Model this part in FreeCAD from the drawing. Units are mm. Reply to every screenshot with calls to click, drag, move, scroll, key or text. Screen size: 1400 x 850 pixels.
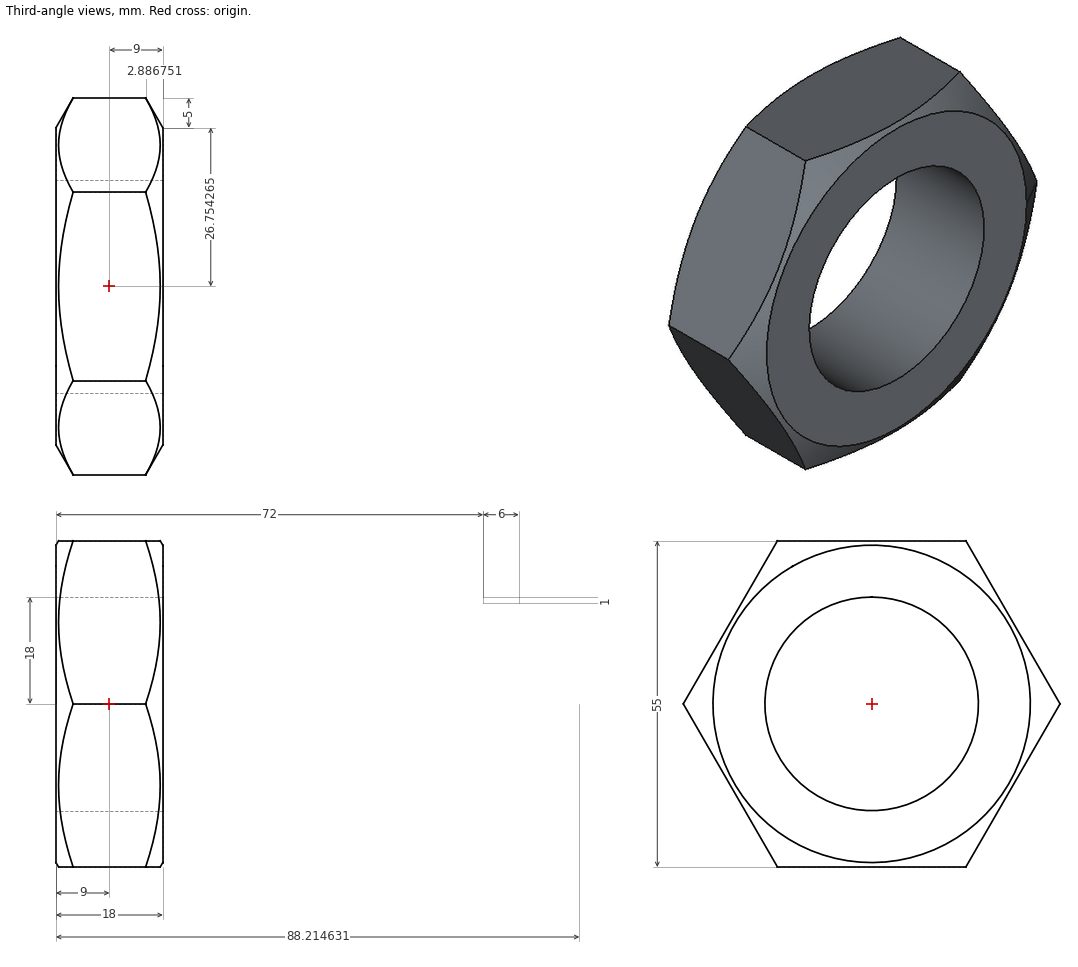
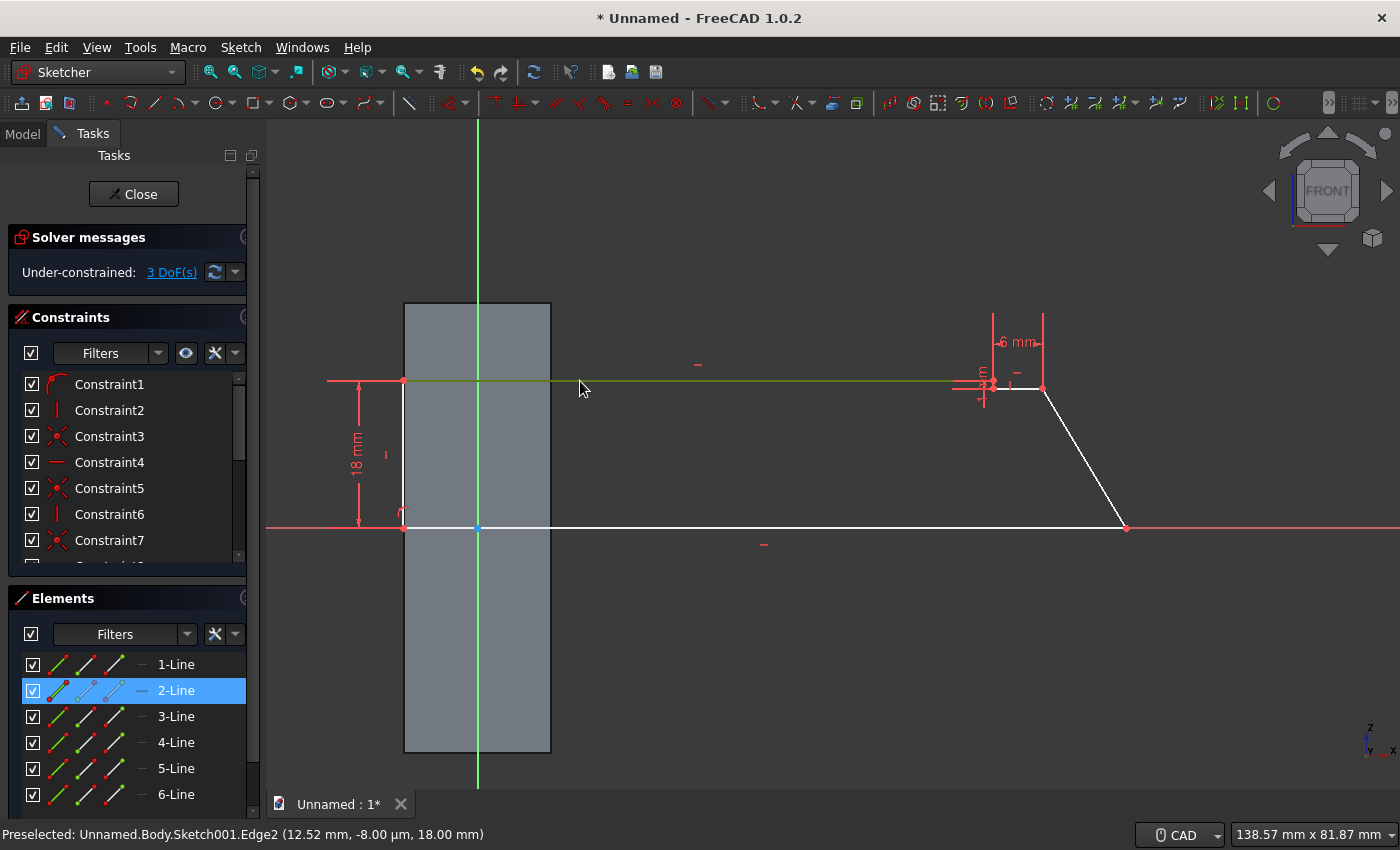
key(l)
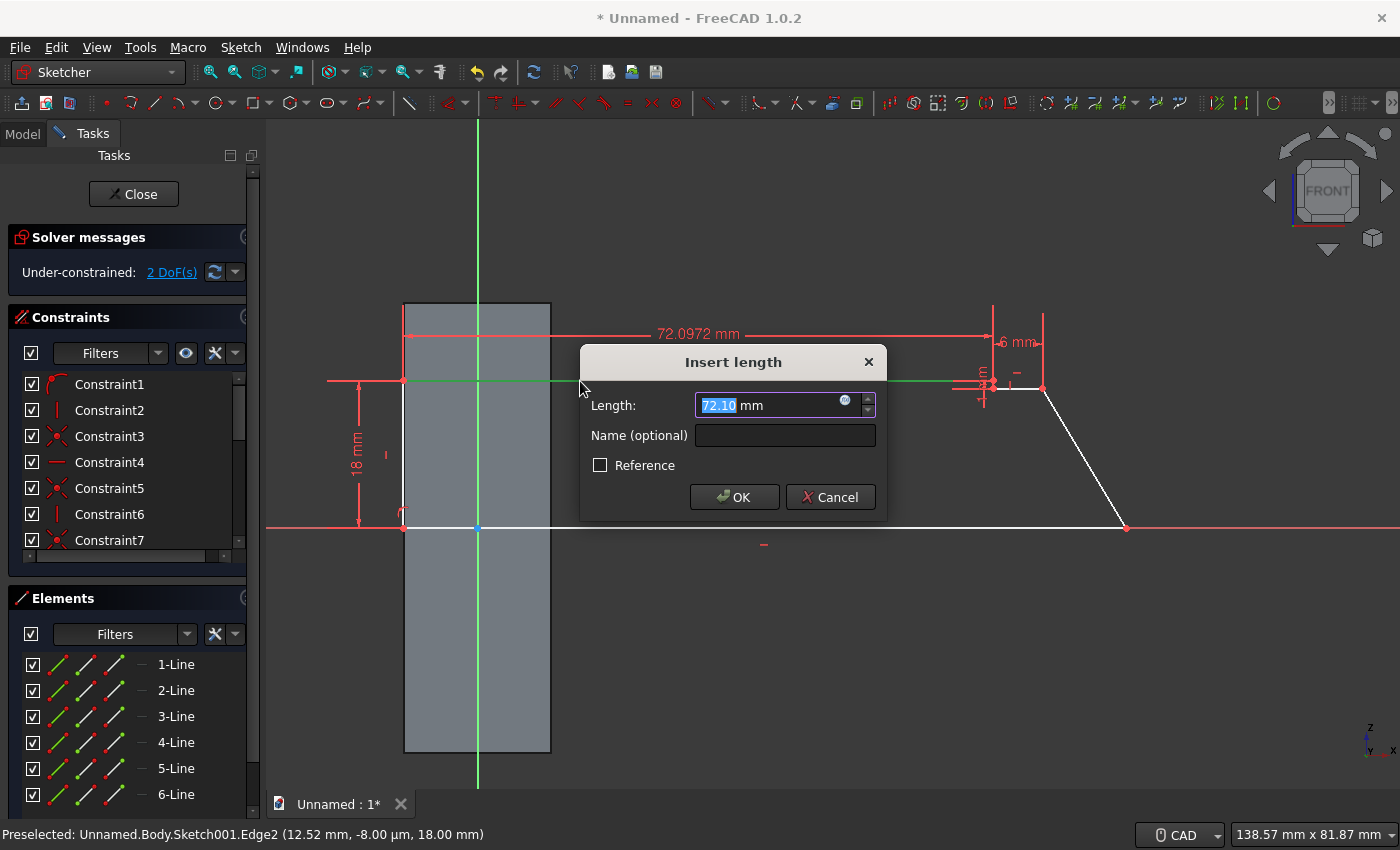
text(72)
key(Return)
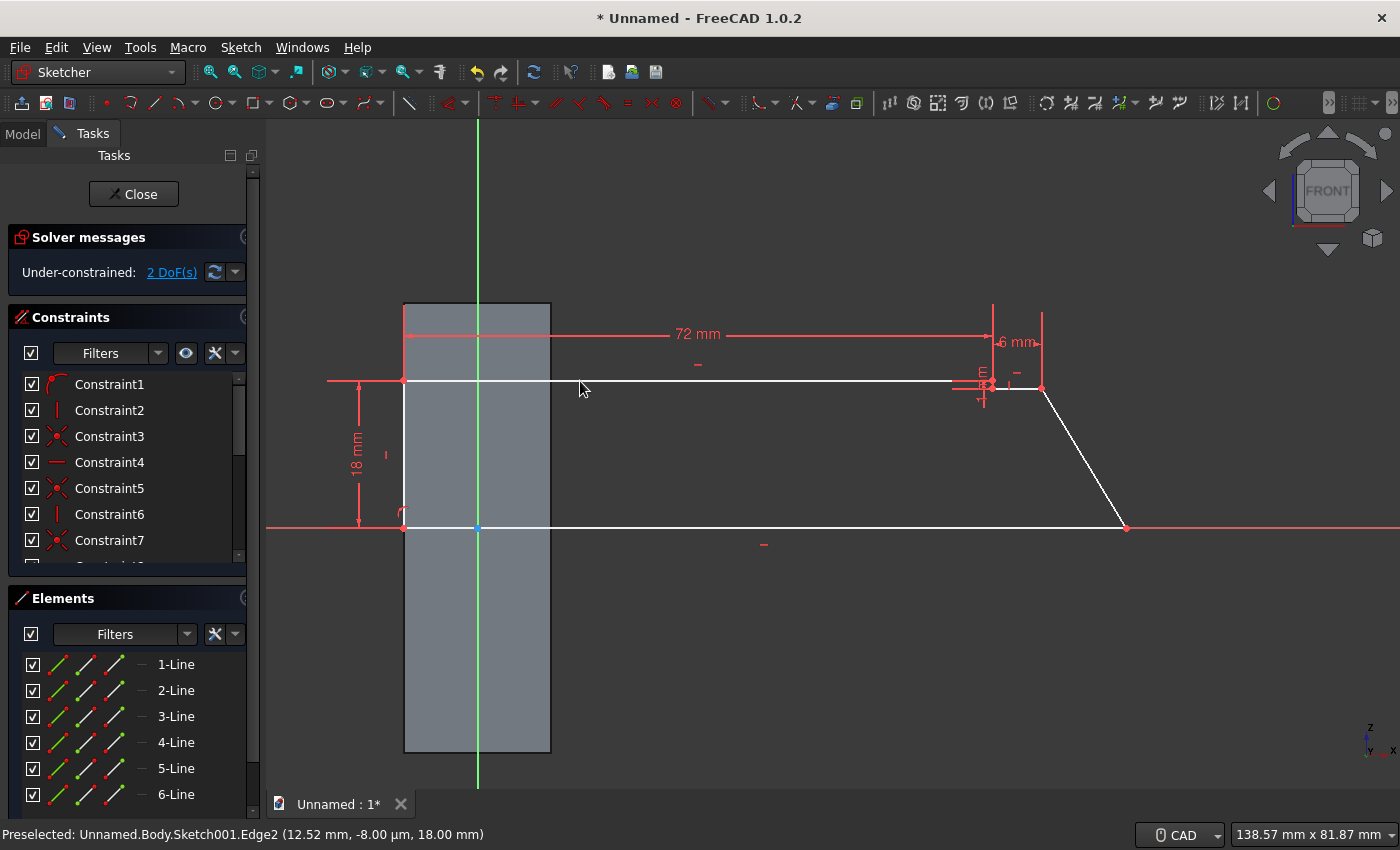
click(404, 528)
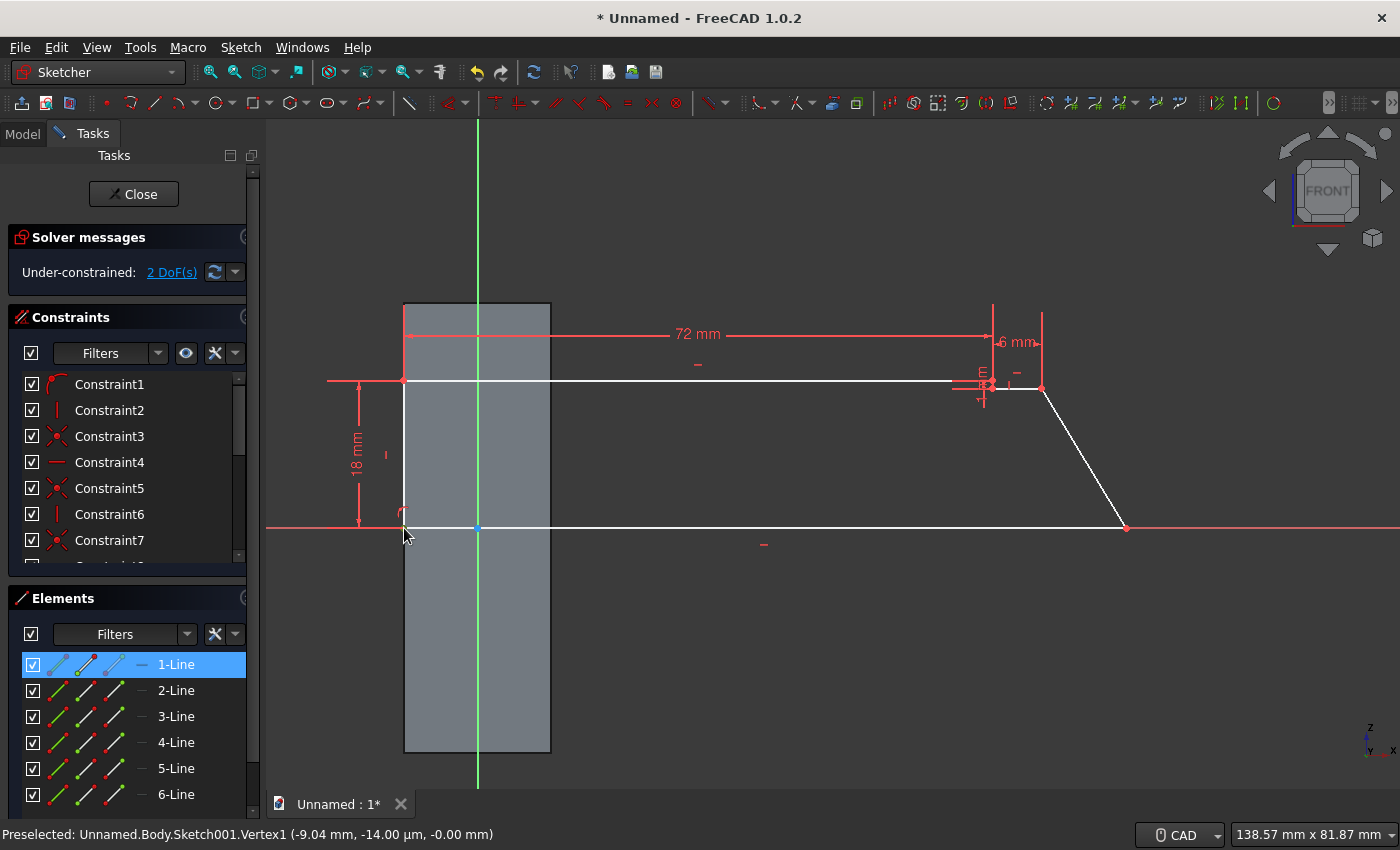
key(l)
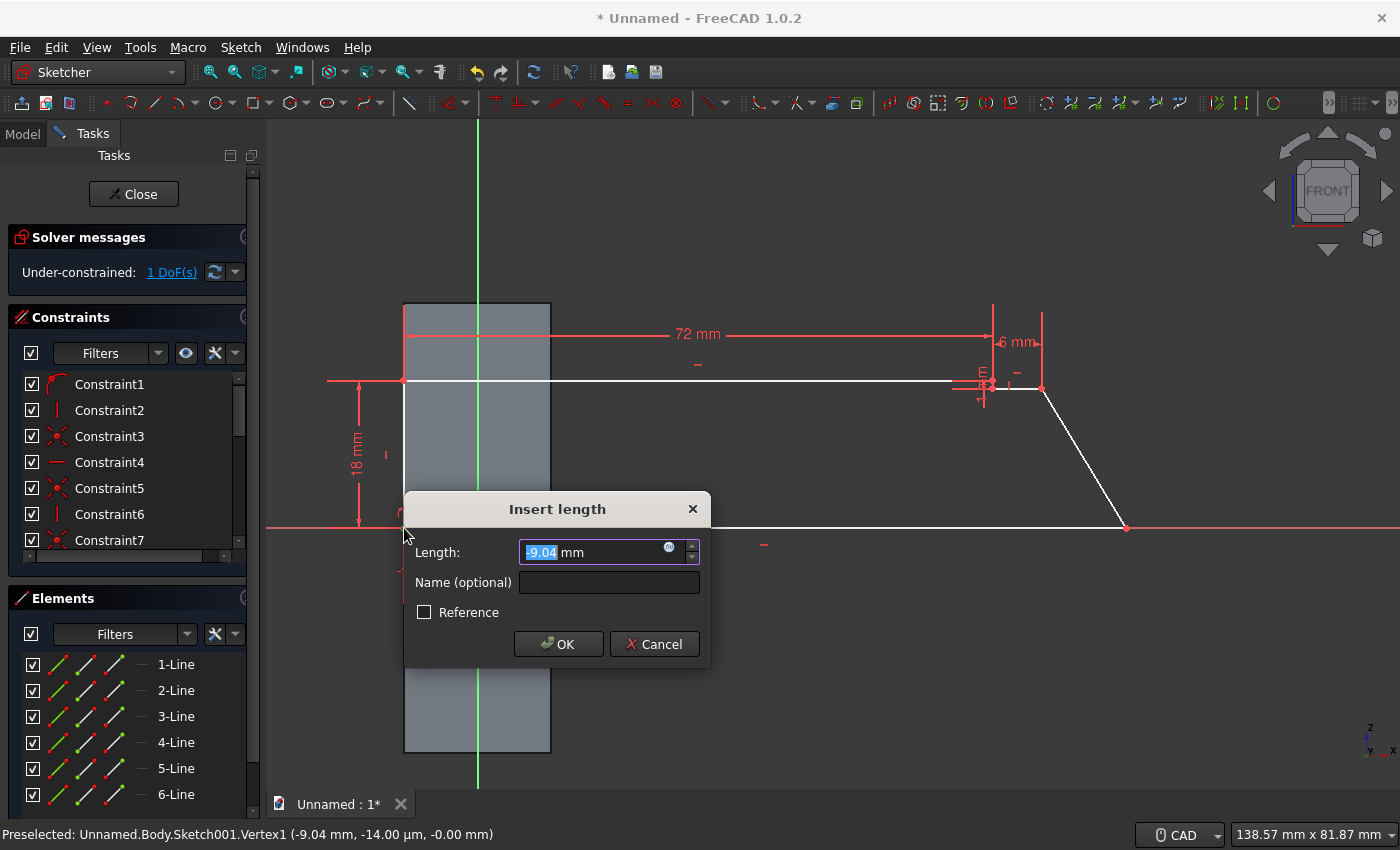
text(-9)
key(Return)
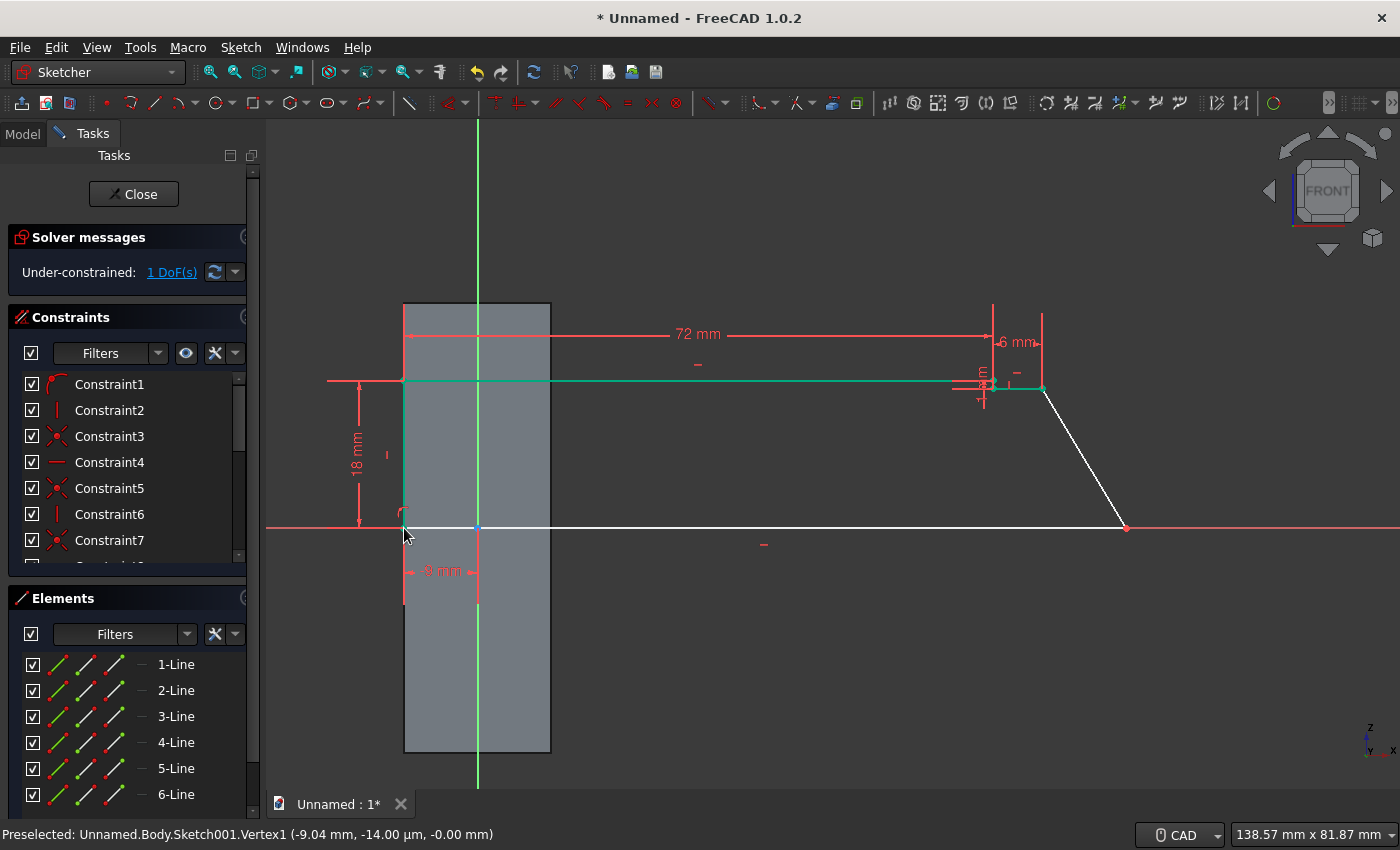
click(909, 528)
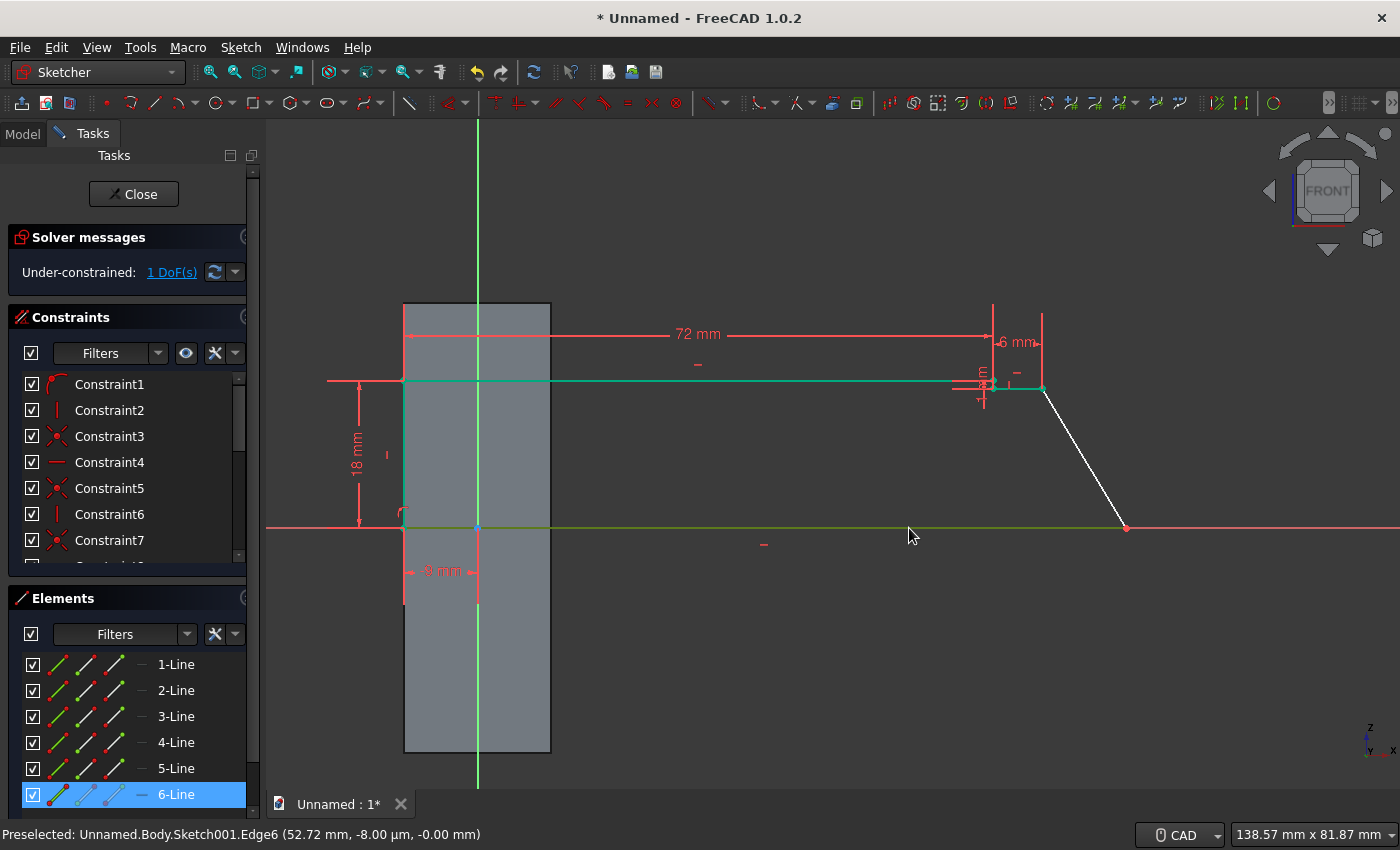
click(468, 104)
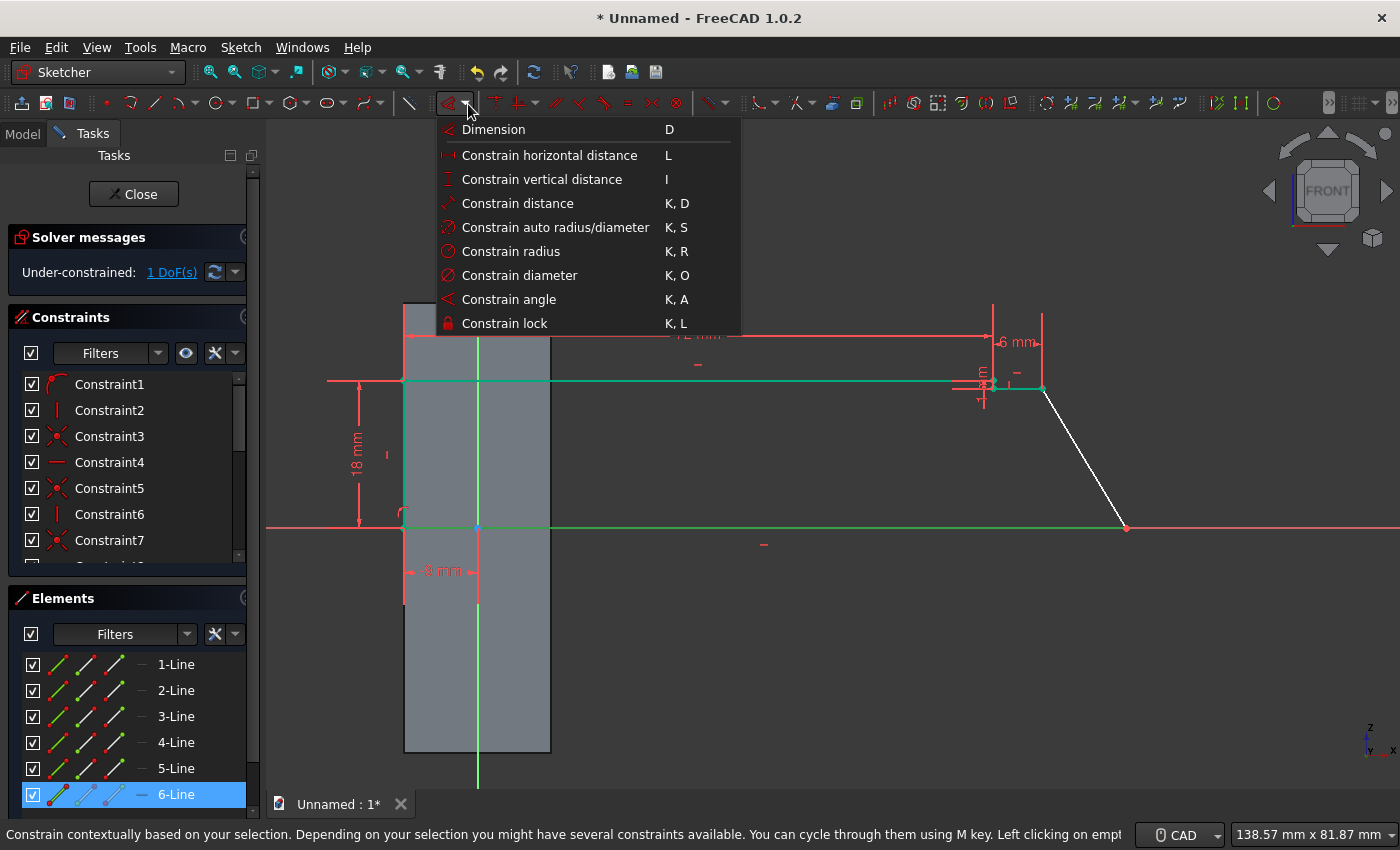
click(589, 155)